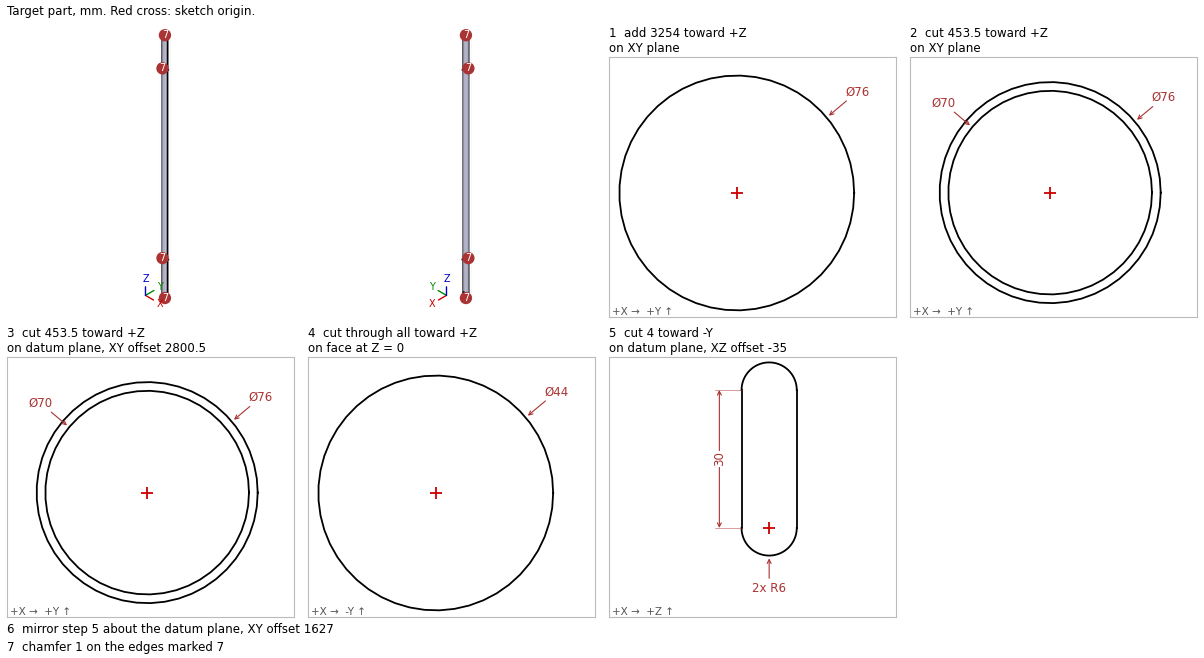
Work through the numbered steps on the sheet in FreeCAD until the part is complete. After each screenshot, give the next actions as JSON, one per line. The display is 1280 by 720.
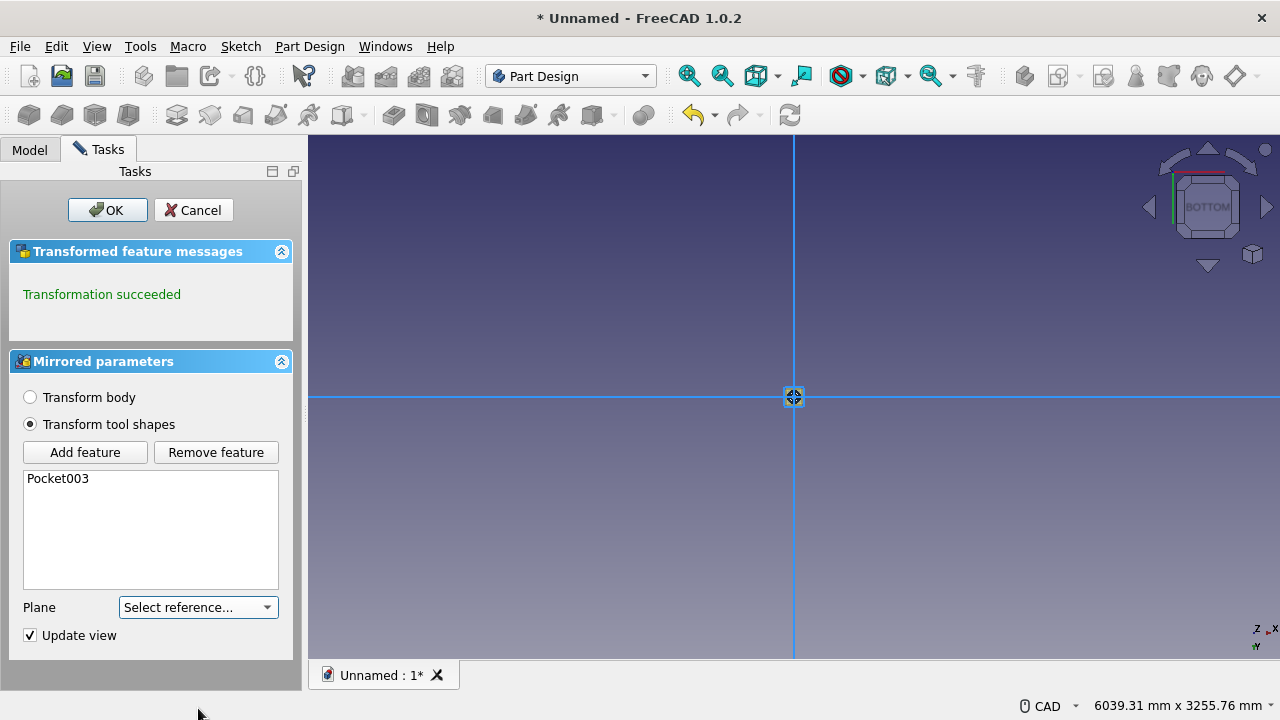
{"action": "left_click", "coordinate": [30, 149]}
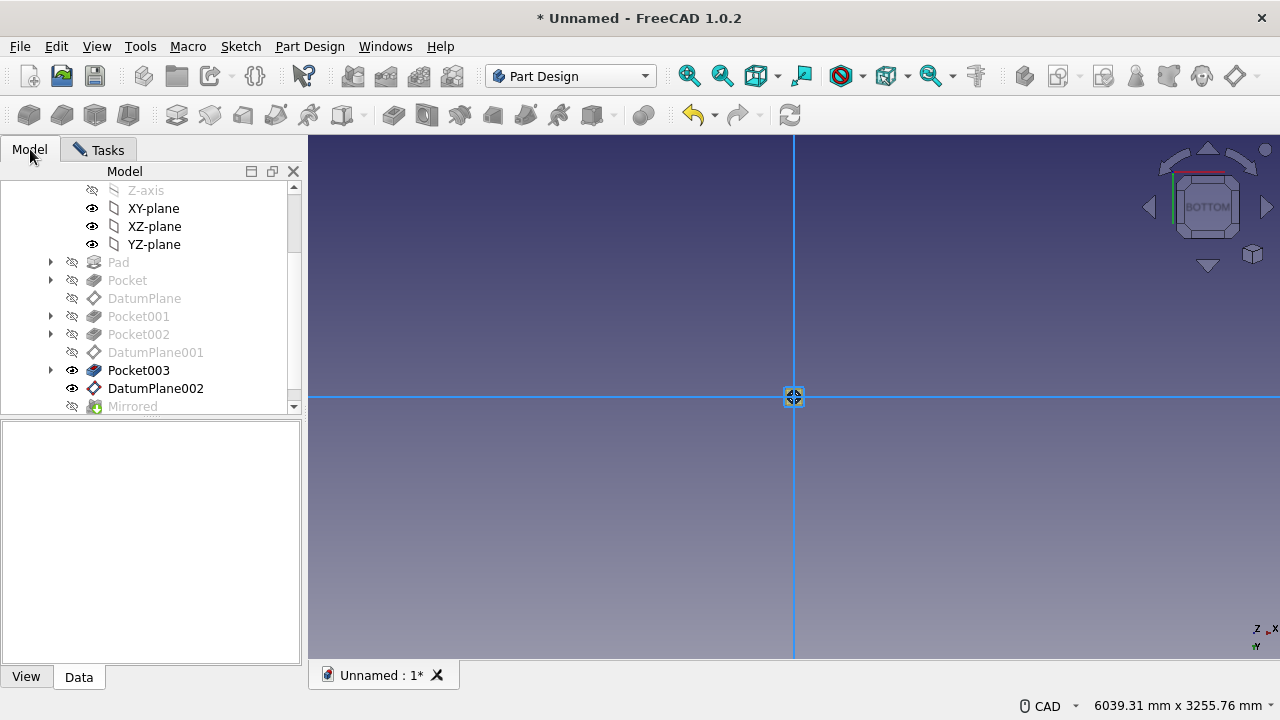
{"action": "left_click", "coordinate": [117, 388]}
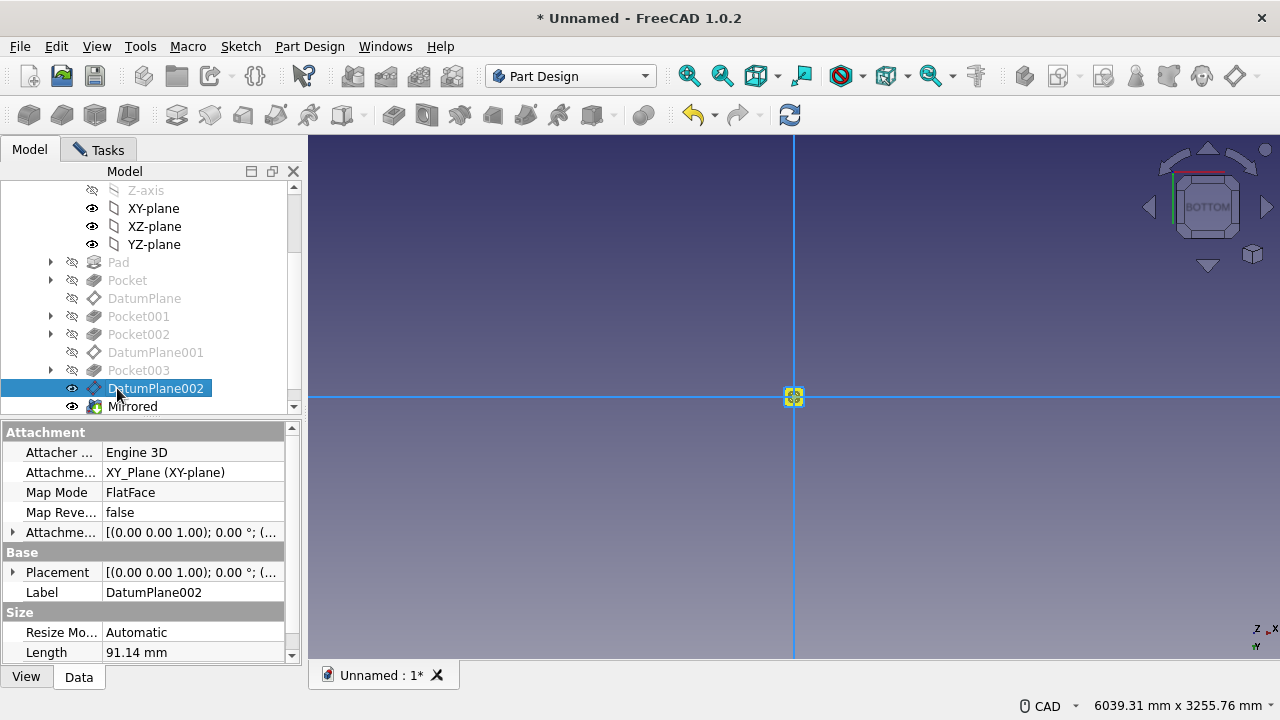
{"action": "left_click", "coordinate": [98, 149]}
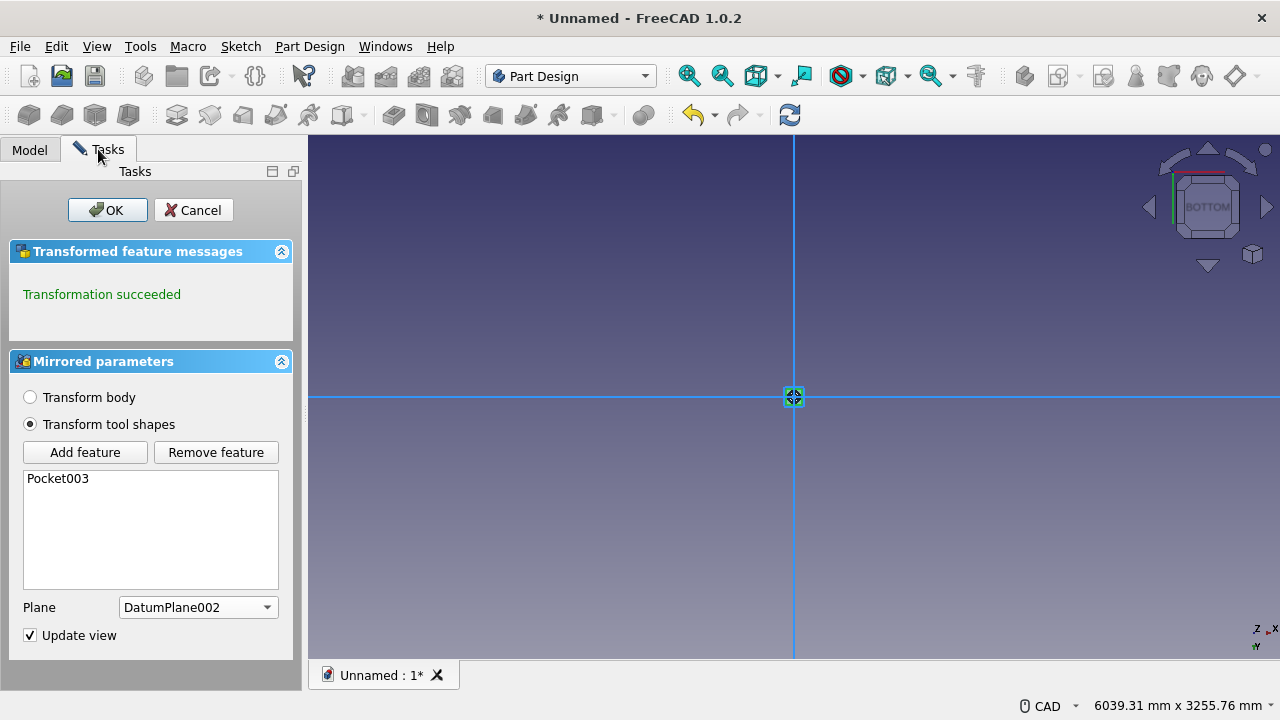
{"action": "left_click", "coordinate": [108, 210]}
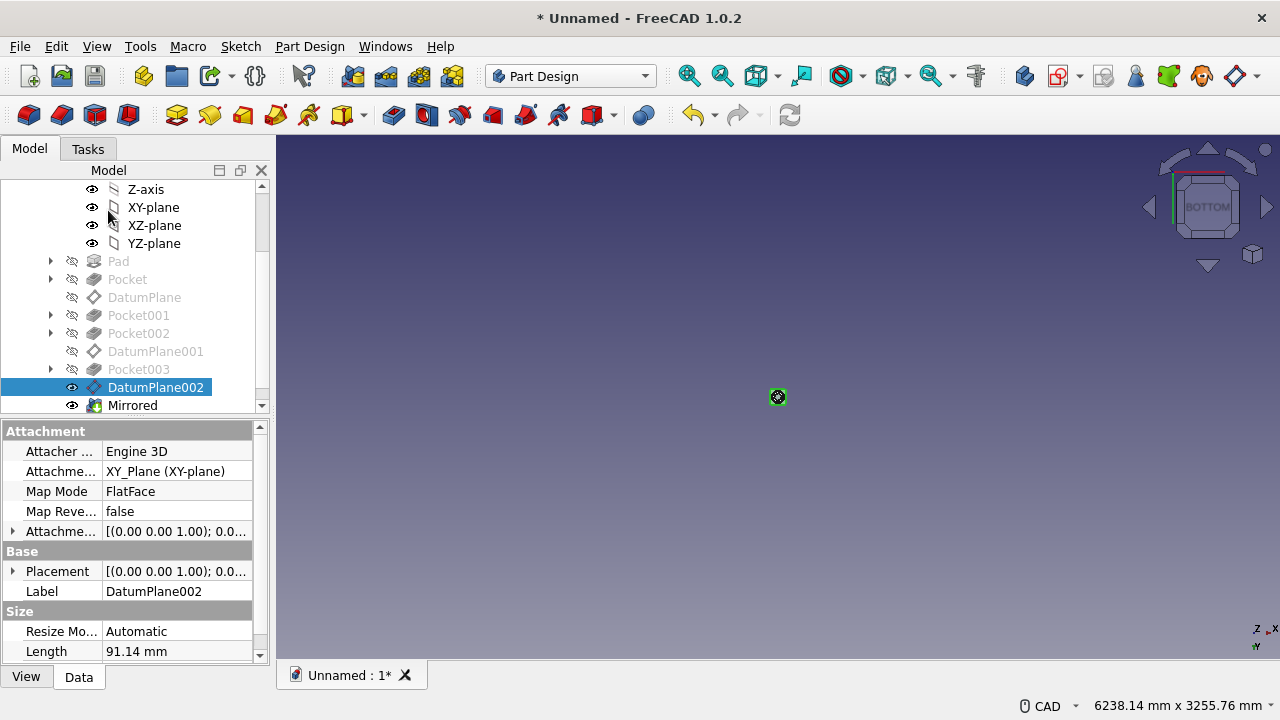
{"action": "left_click", "coordinate": [117, 387]}
{"action": "key", "text": "space"}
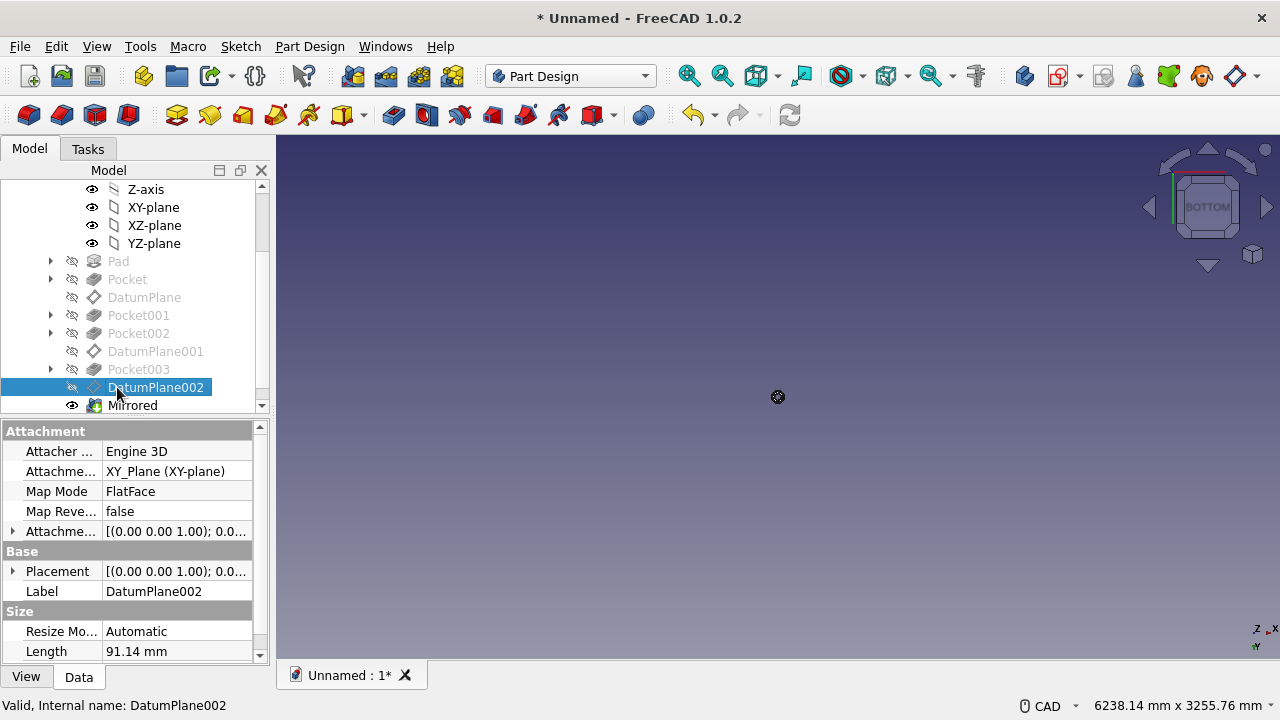
{"action": "left_click", "coordinate": [690, 76]}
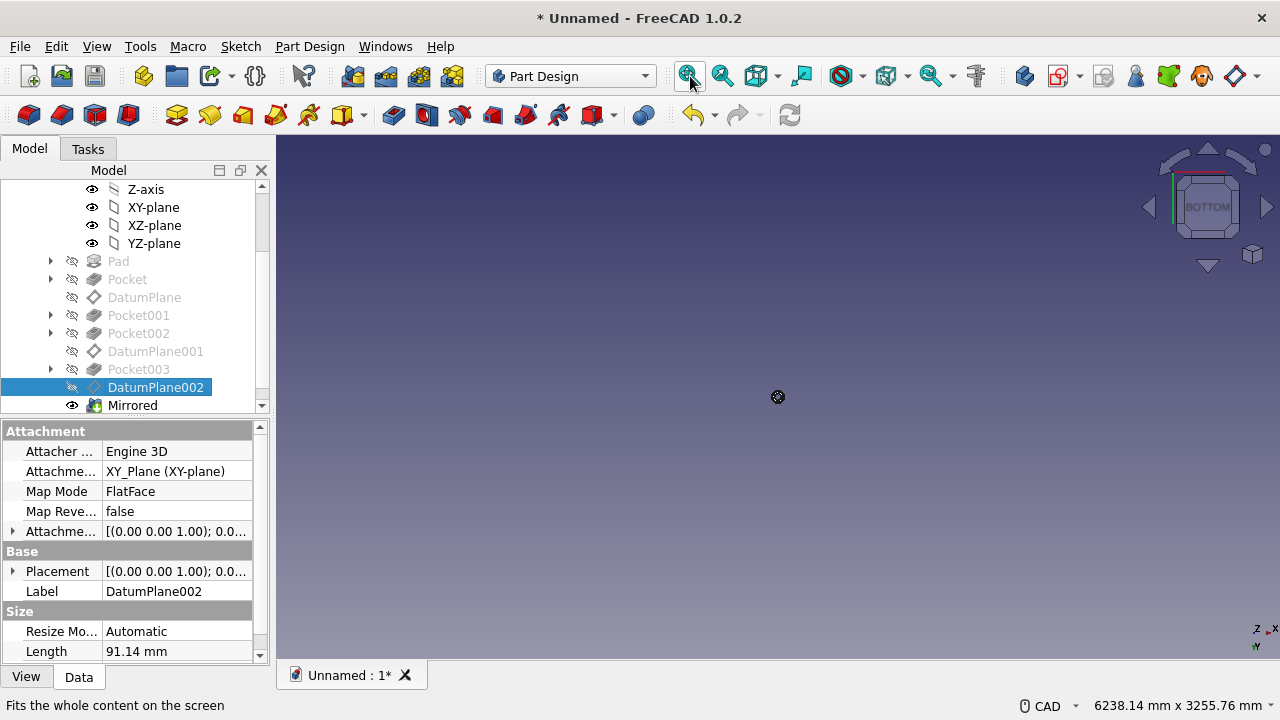
{"action": "left_click", "coordinate": [772, 396]}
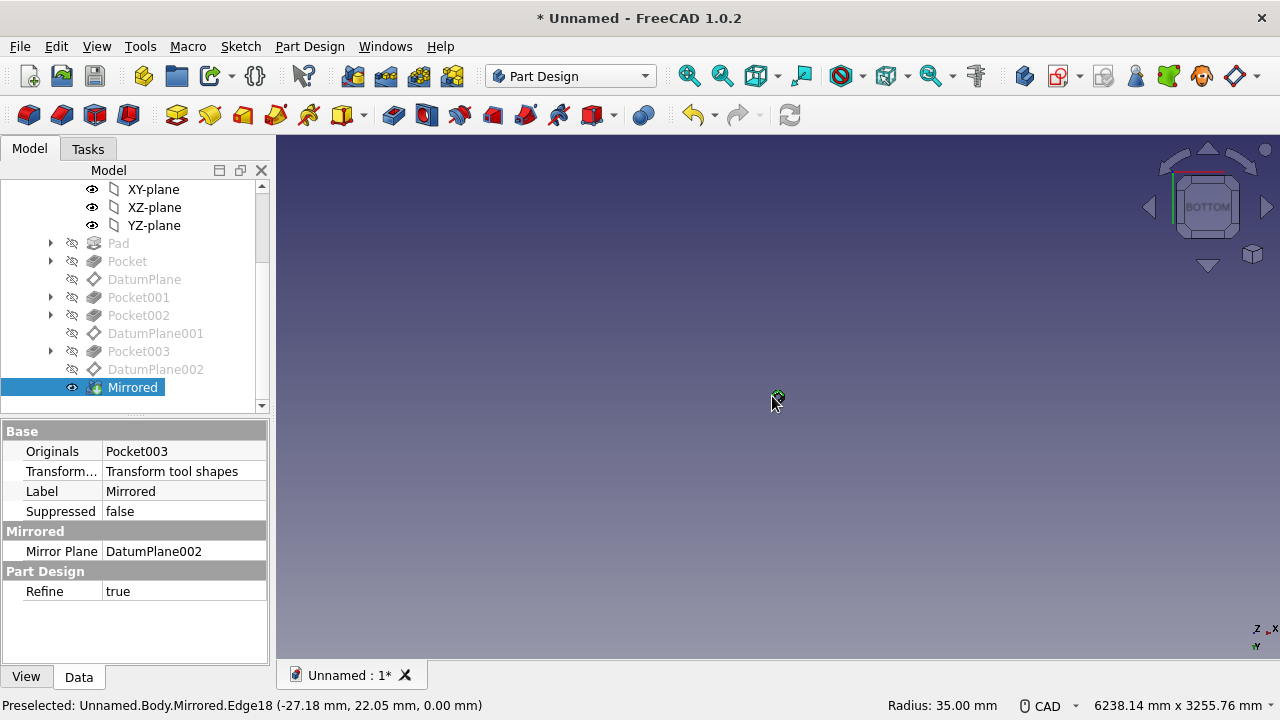
{"action": "key", "text": "0"}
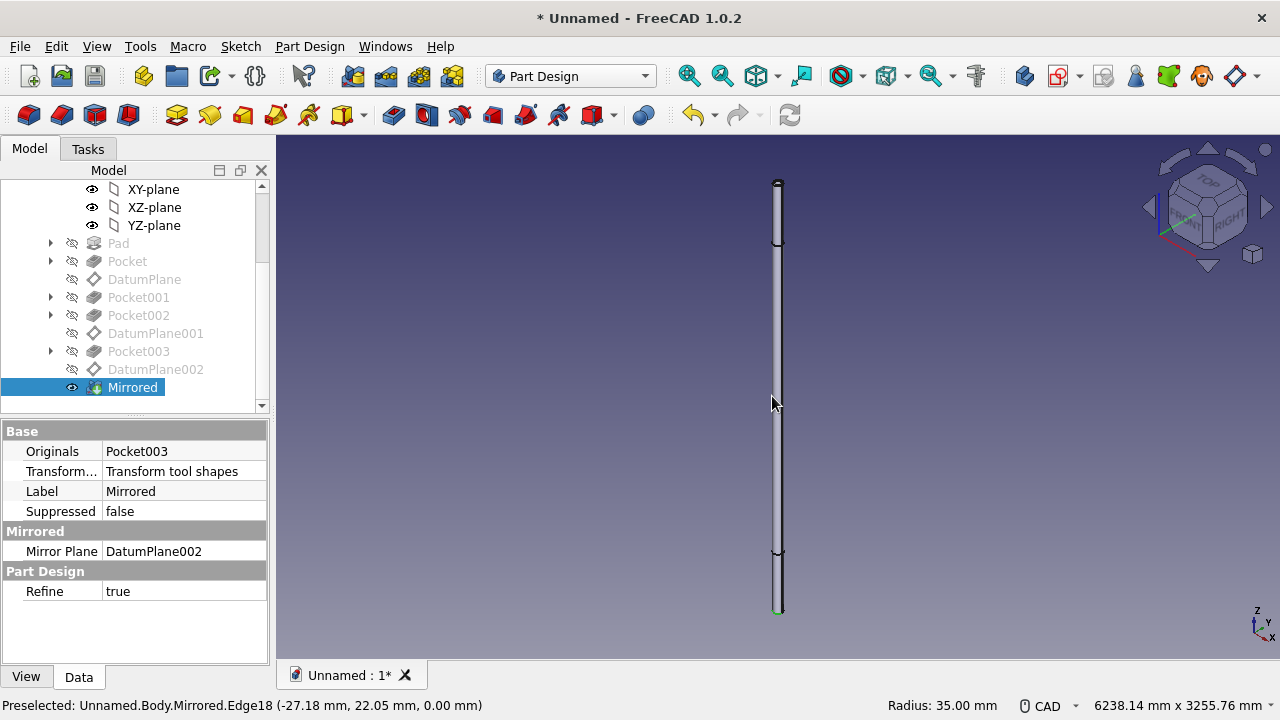
{"action": "left_click", "coordinate": [773, 243], "text": "ctrl"}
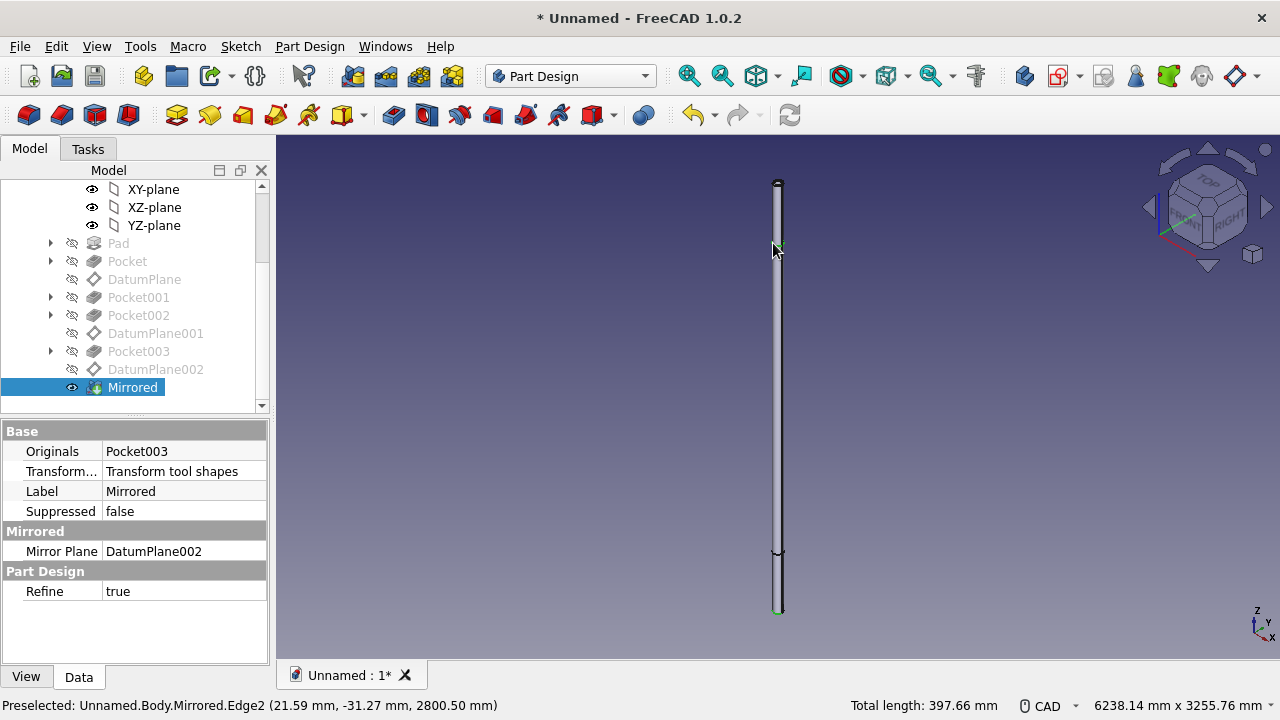
{"action": "left_click", "coordinate": [772, 182], "text": "ctrl"}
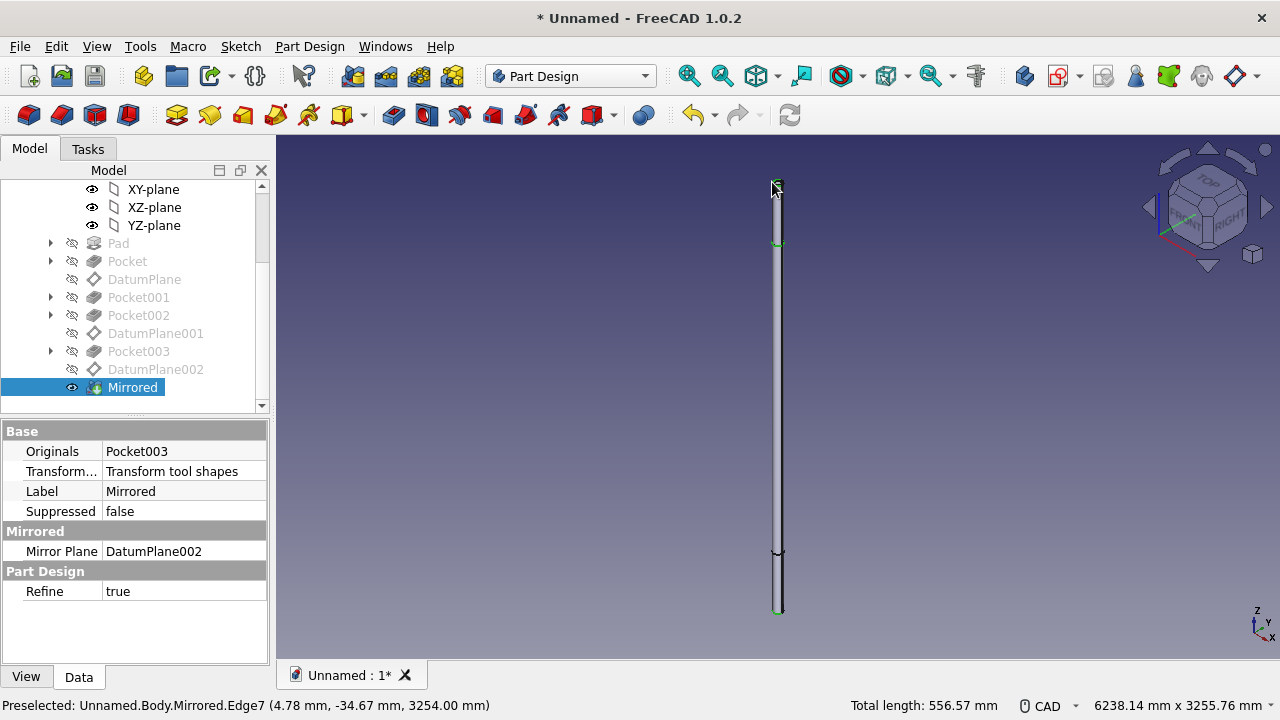
{"action": "key", "text": "2"}